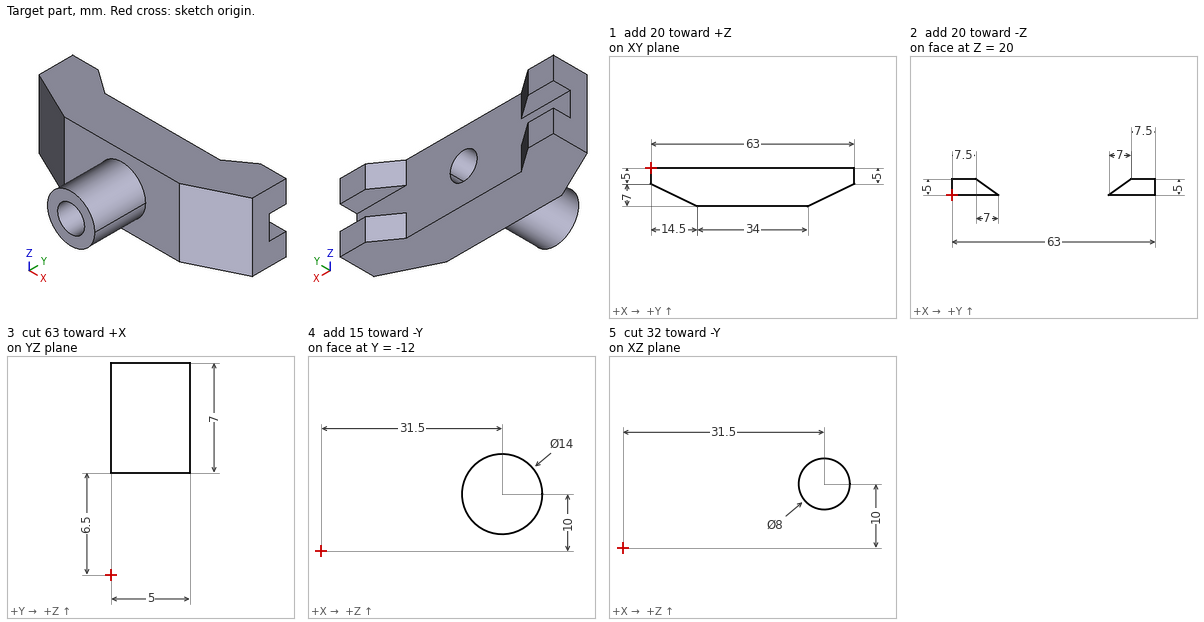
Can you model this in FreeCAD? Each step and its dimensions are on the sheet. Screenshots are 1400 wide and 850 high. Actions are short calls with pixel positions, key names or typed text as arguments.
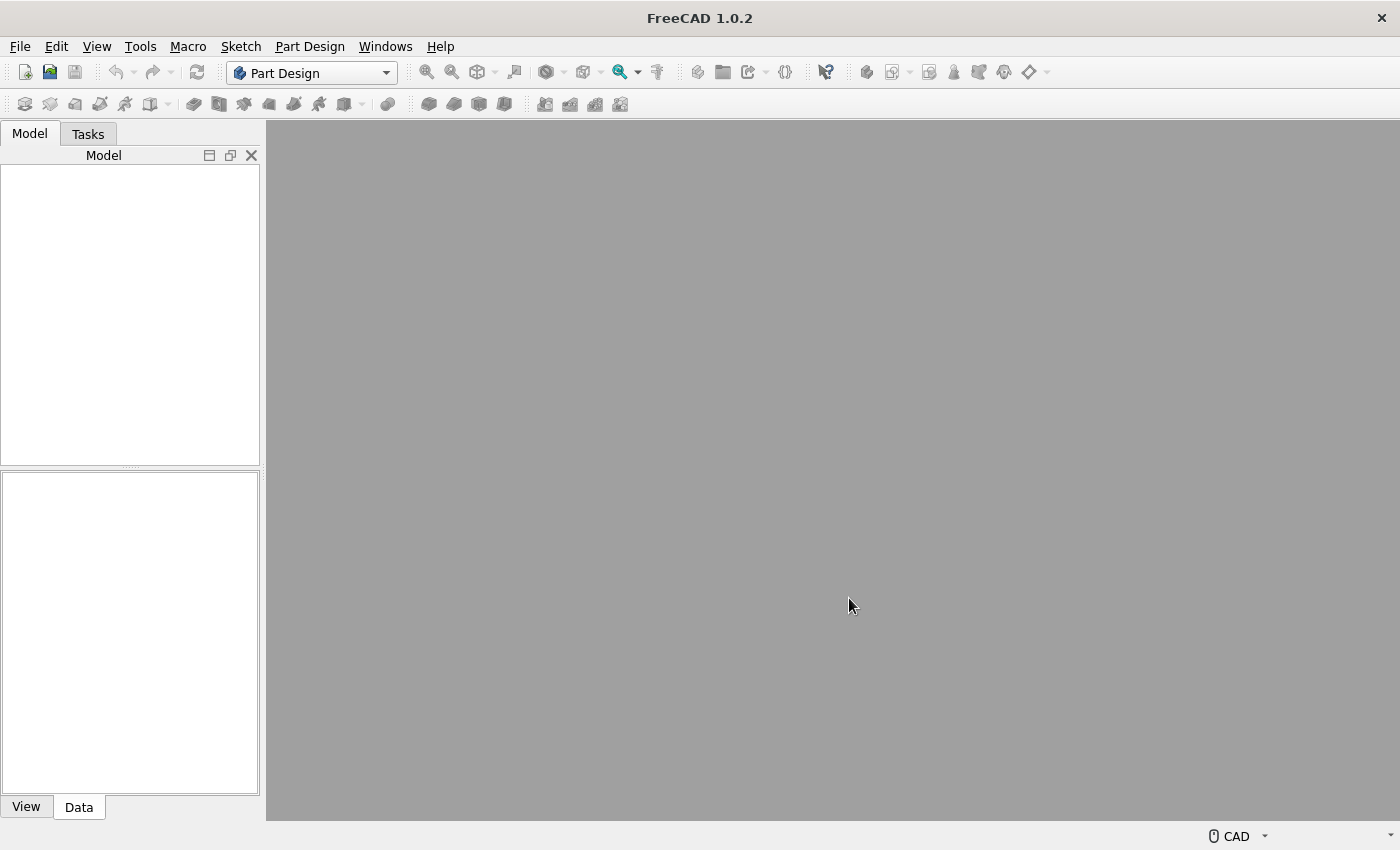
click(25, 72)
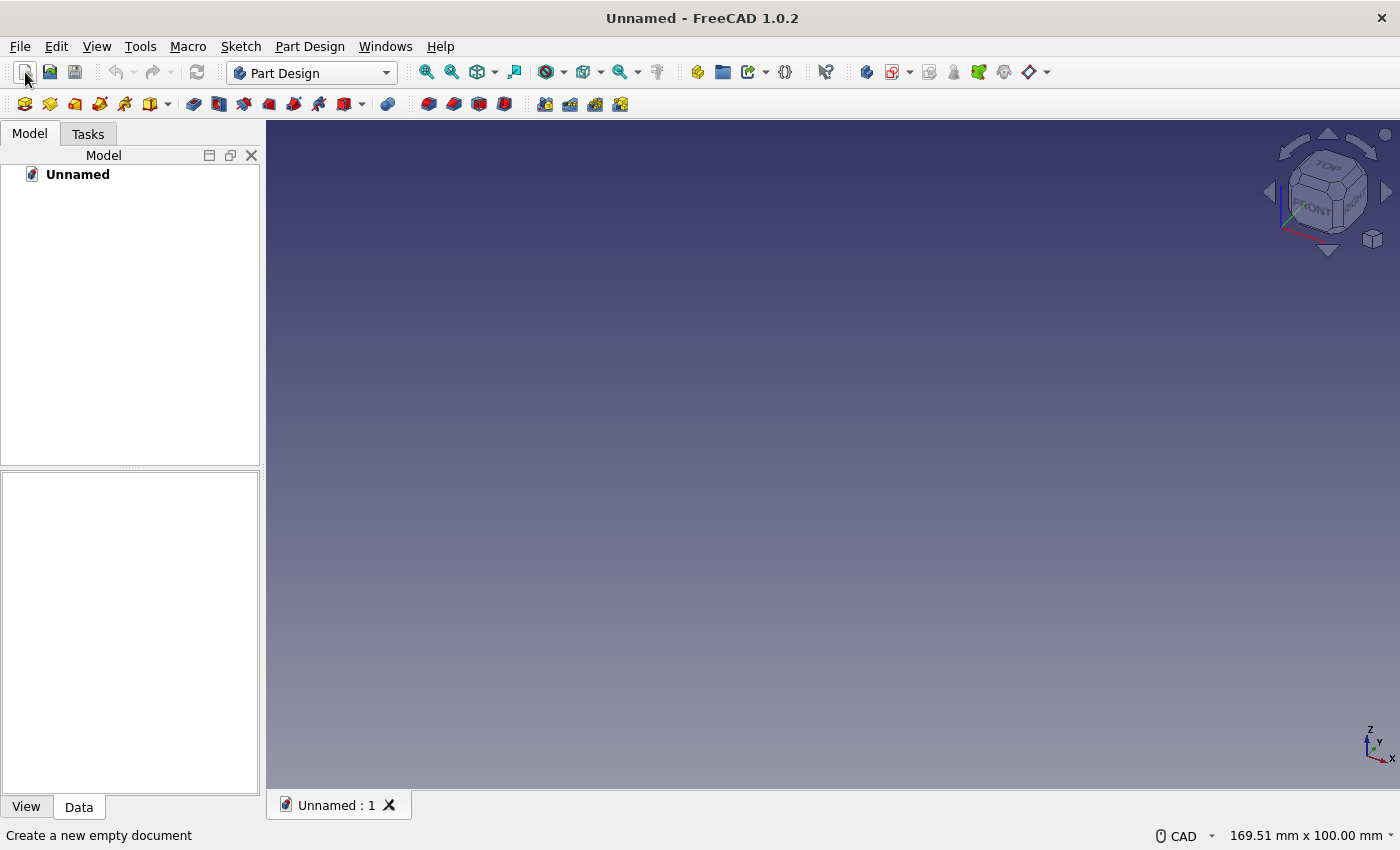
click(892, 72)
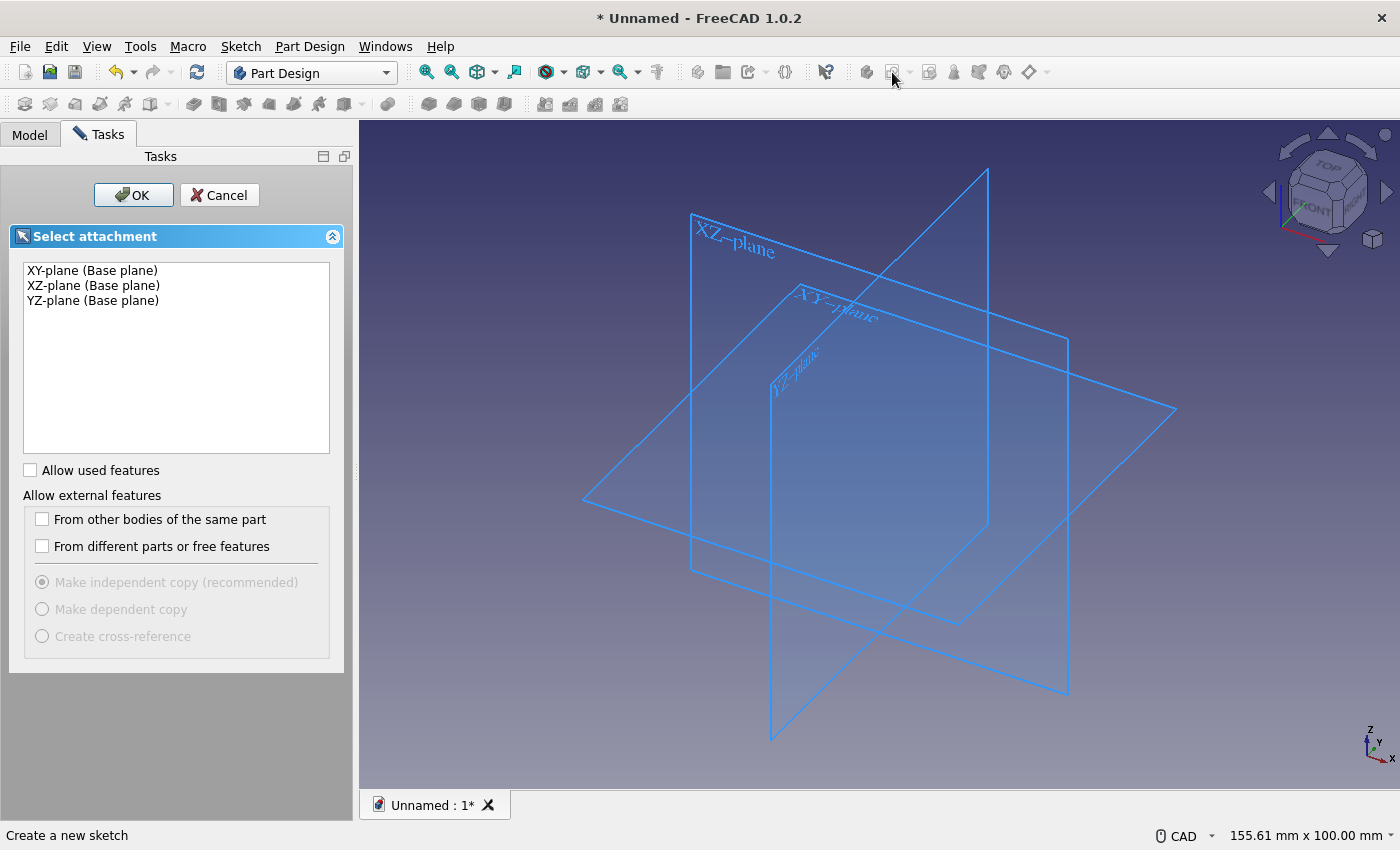
click(84, 270)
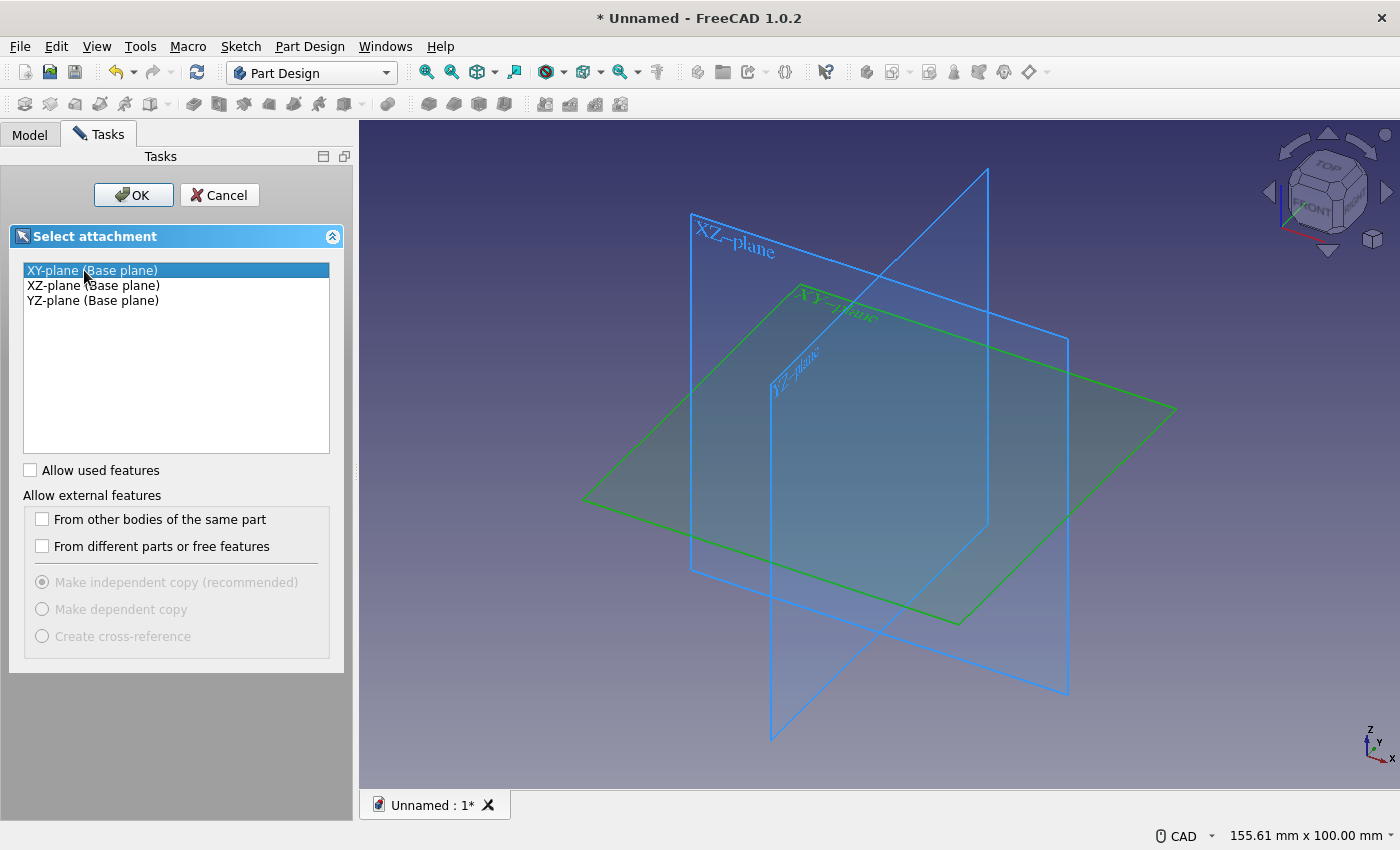
click(134, 195)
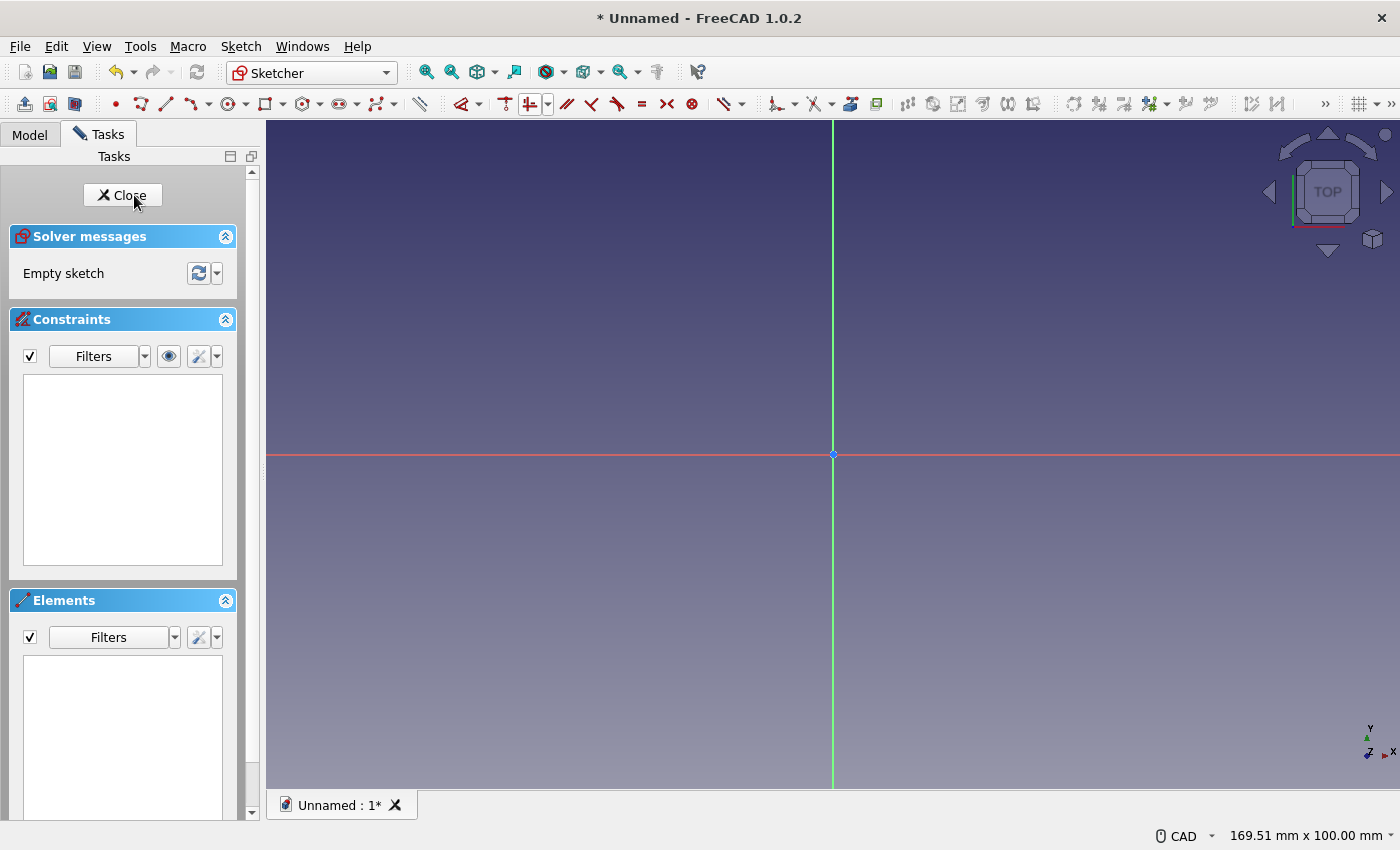
scroll(294, 273, down, 1)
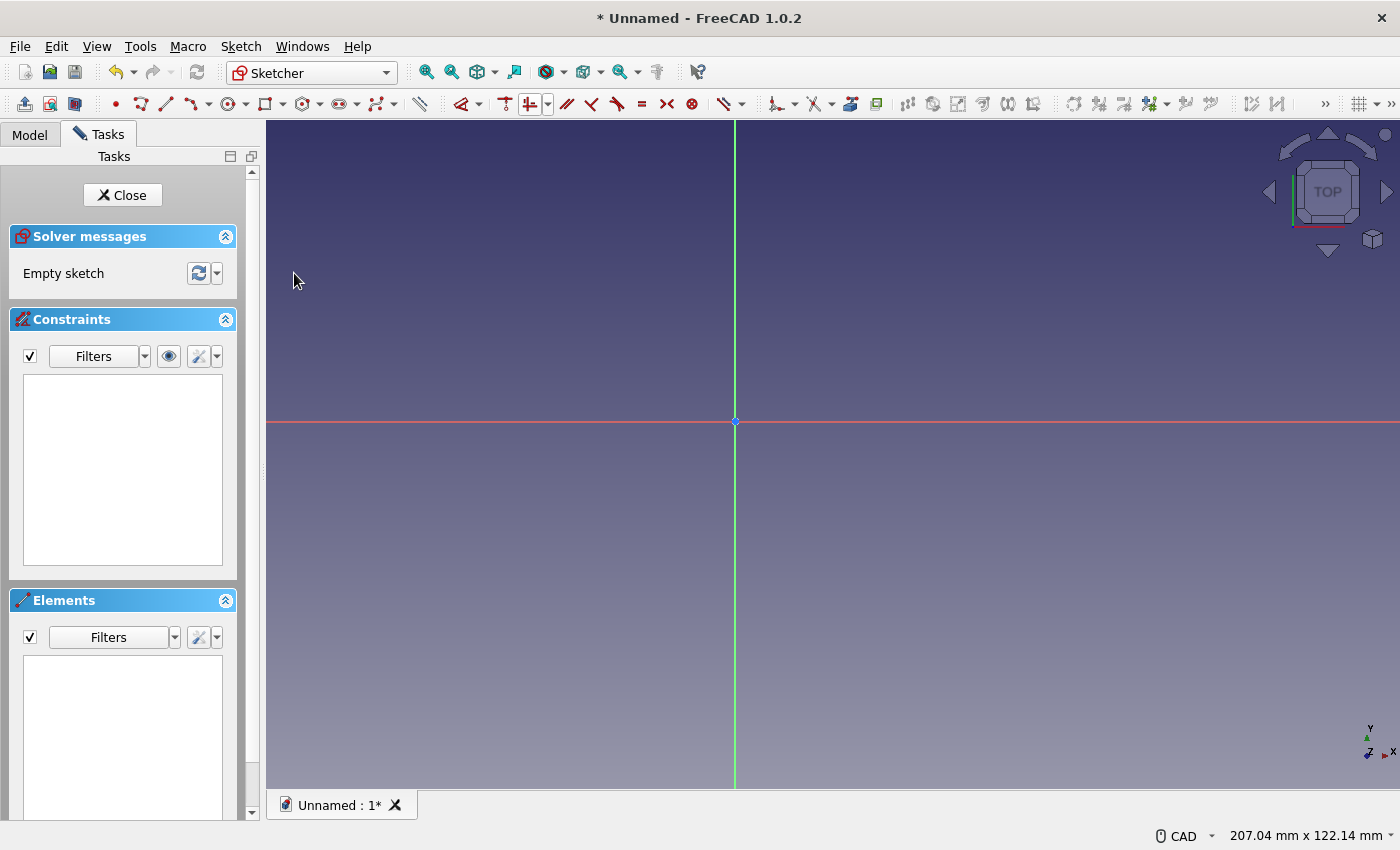
scroll(1082, 455, up, 3)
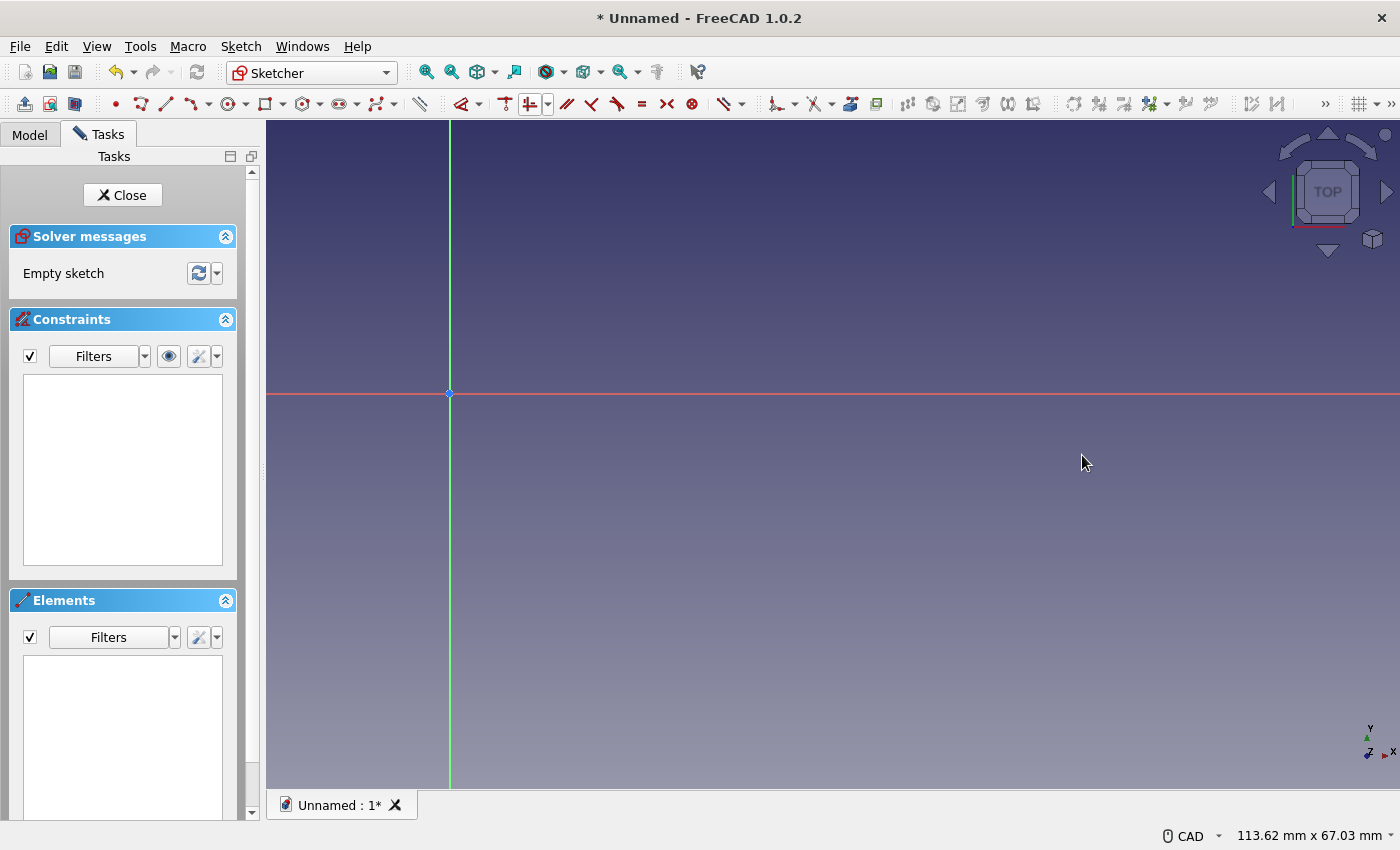
click(141, 104)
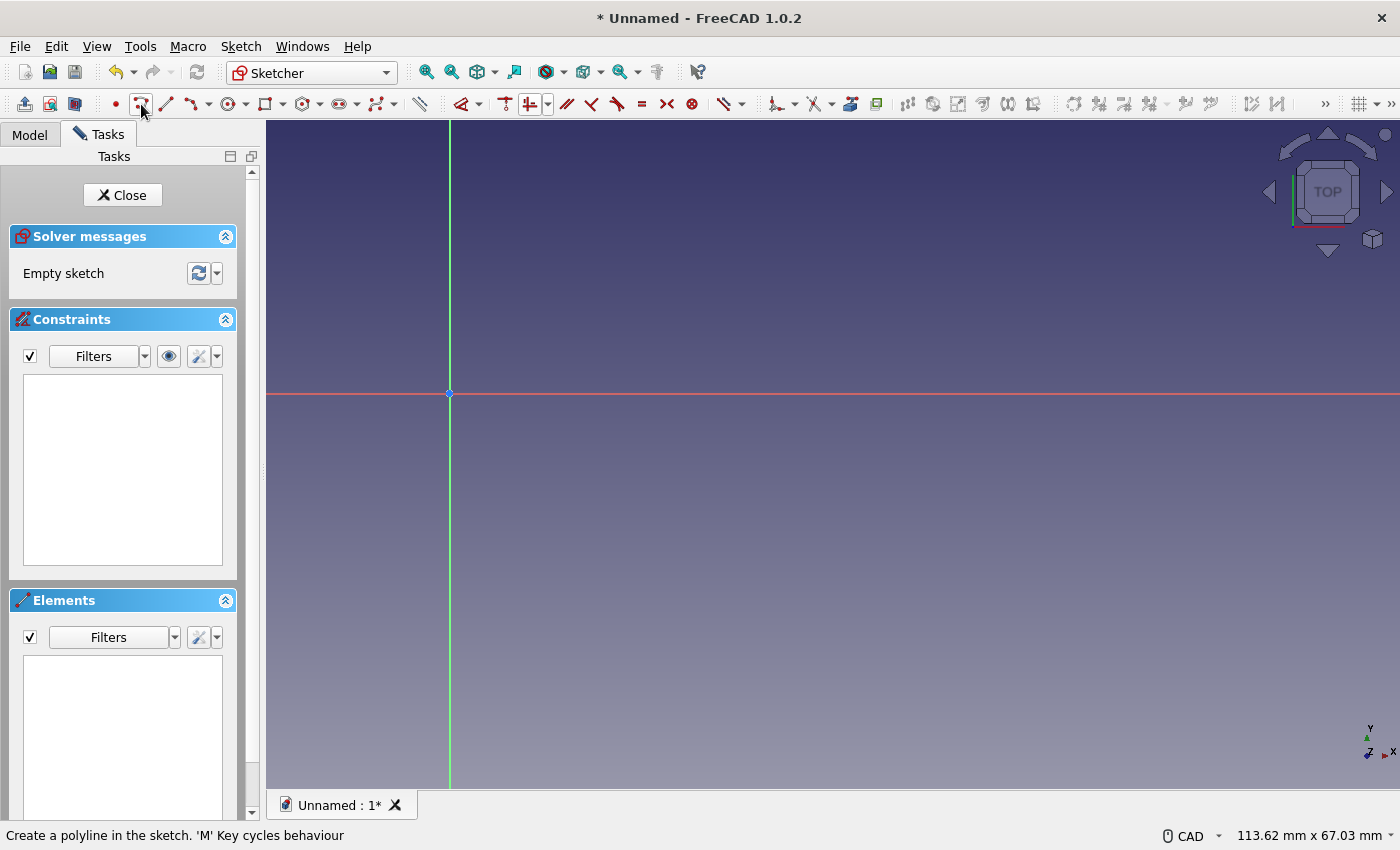
click(450, 394)
click(459, 444)
click(594, 514)
click(934, 514)
click(1078, 444)
click(1078, 403)
click(450, 394)
key(Escape)
key(Escape)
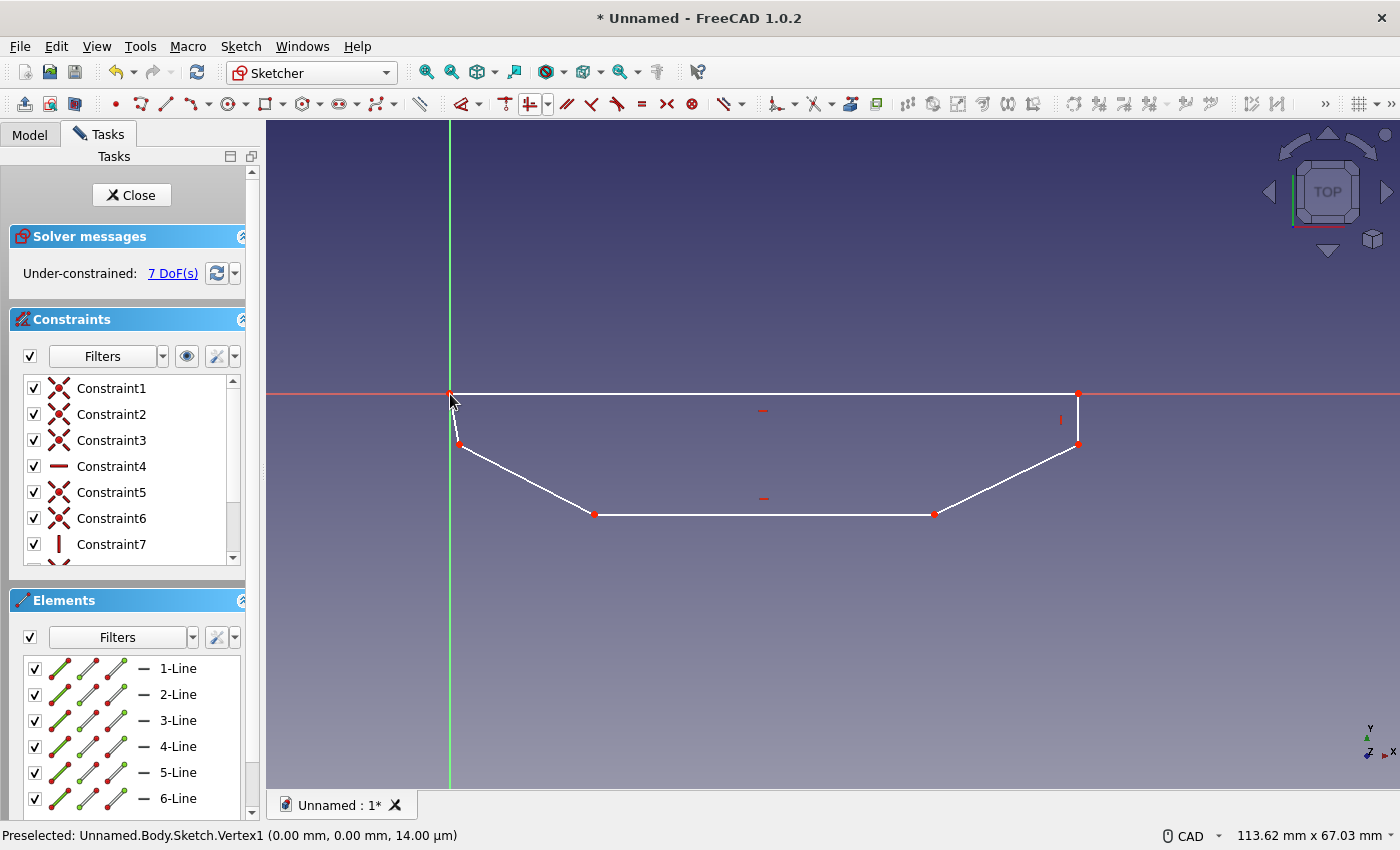
click(452, 409)